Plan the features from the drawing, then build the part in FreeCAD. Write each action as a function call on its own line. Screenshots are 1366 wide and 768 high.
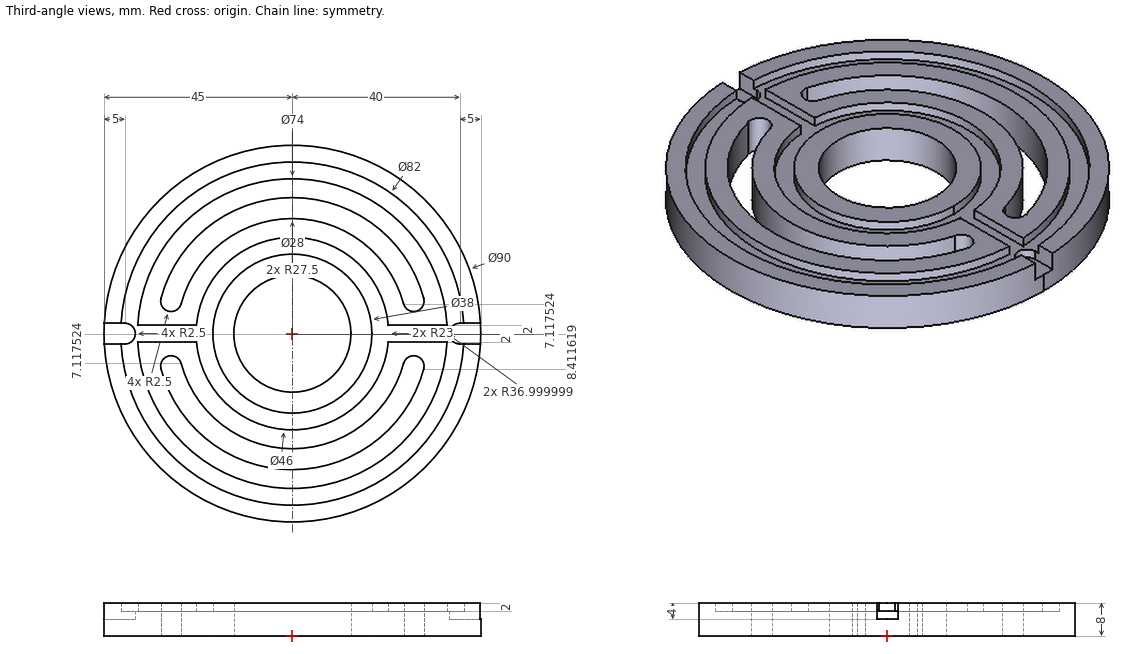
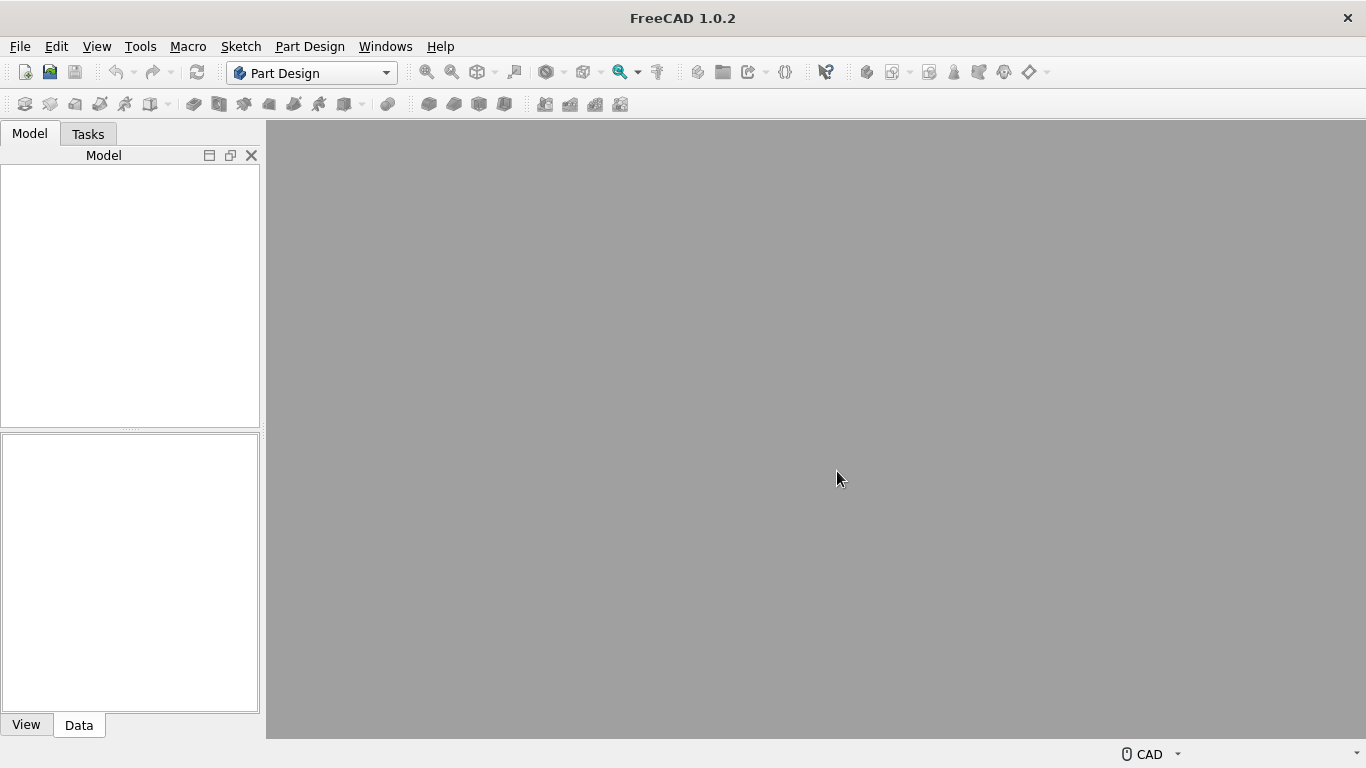
key(ctrl+n)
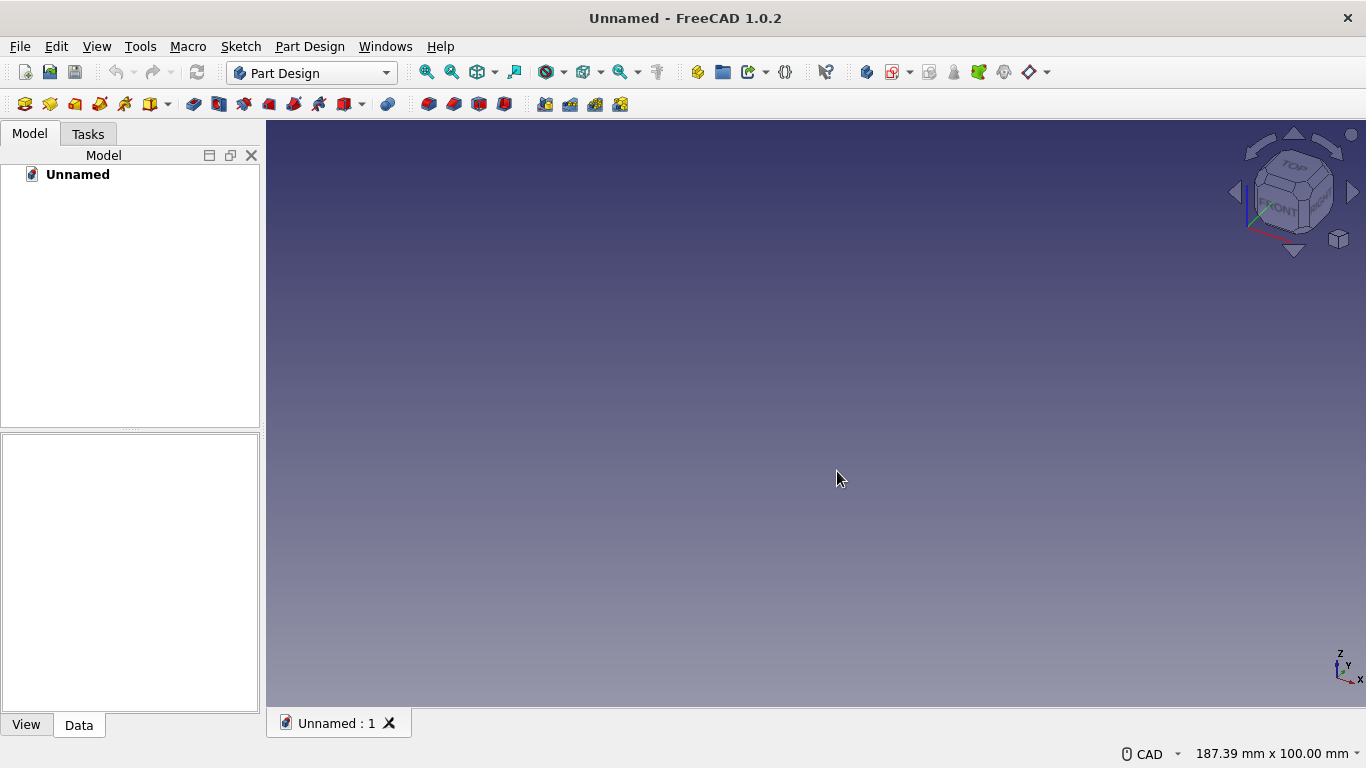
click(892, 72)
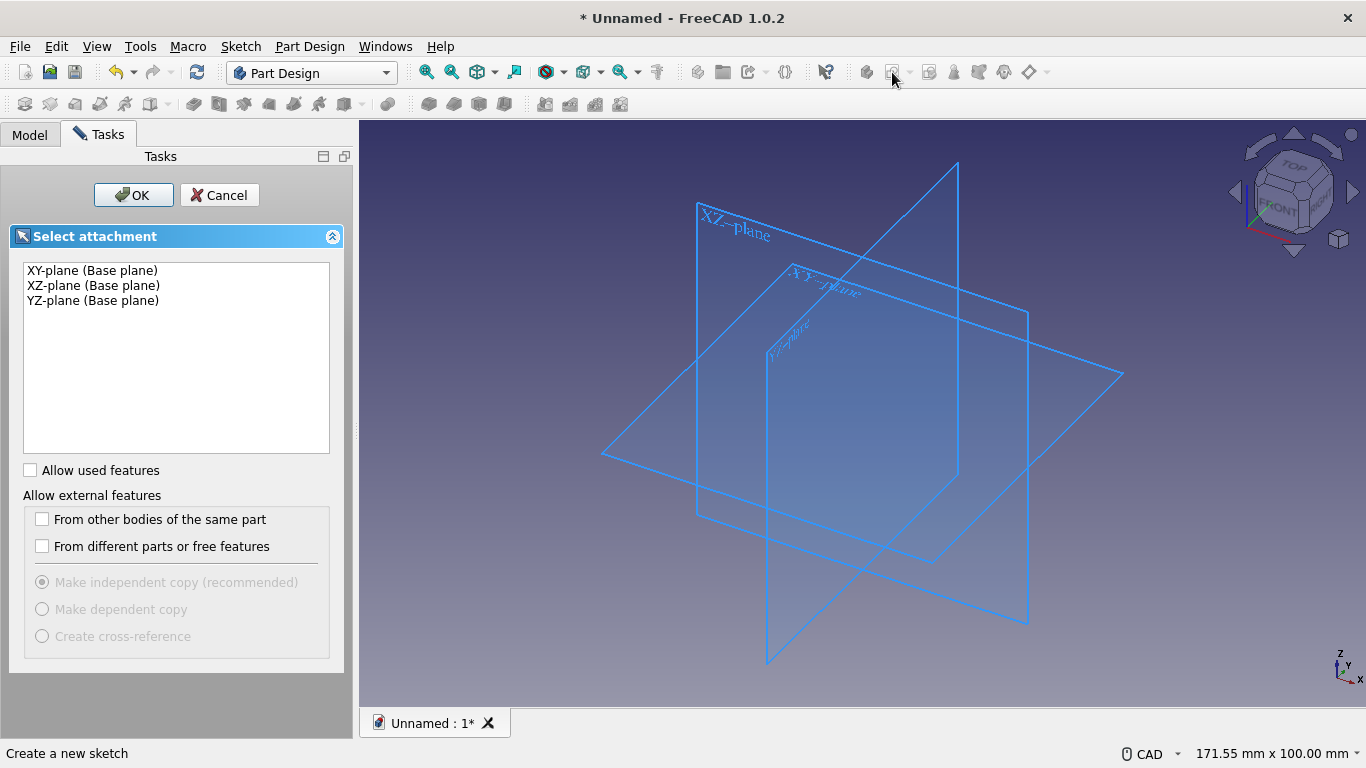
click(84, 270)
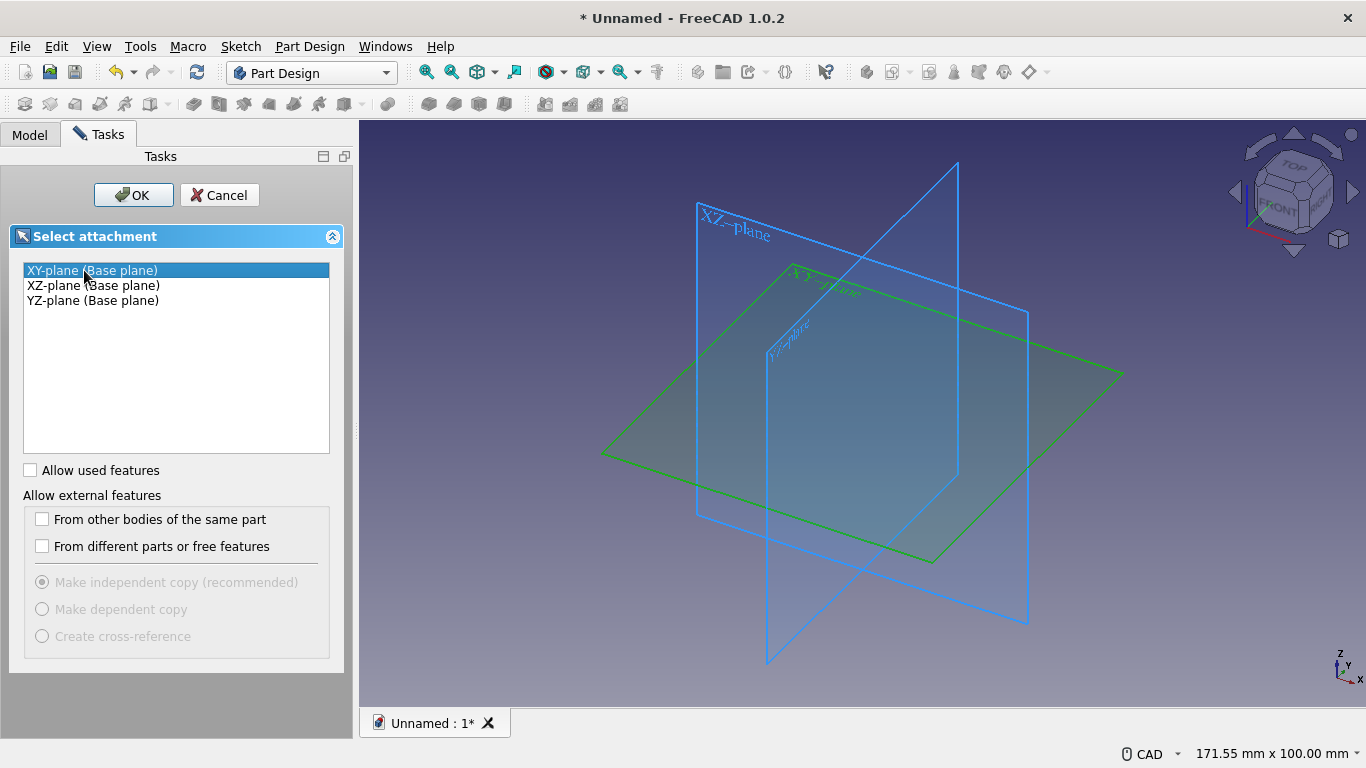
click(134, 195)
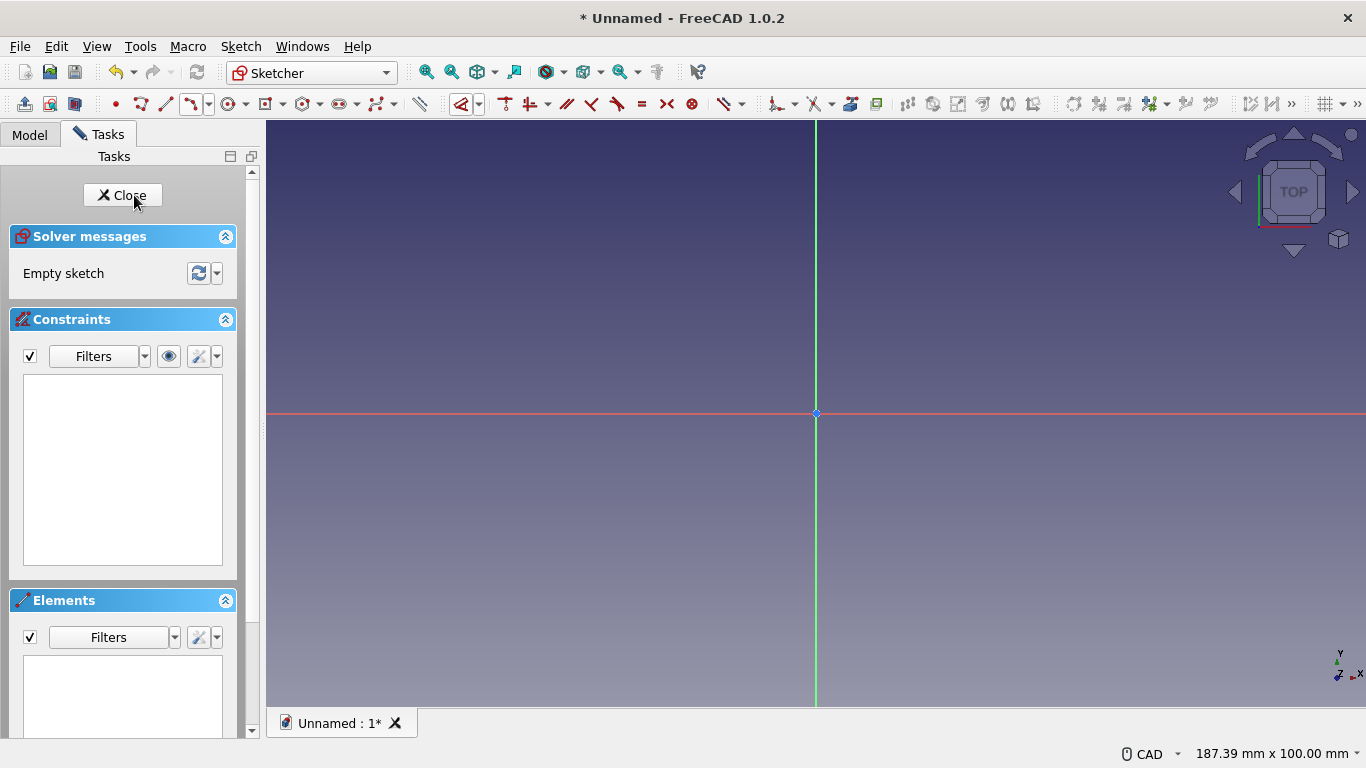
scroll(608, 414, down, 2)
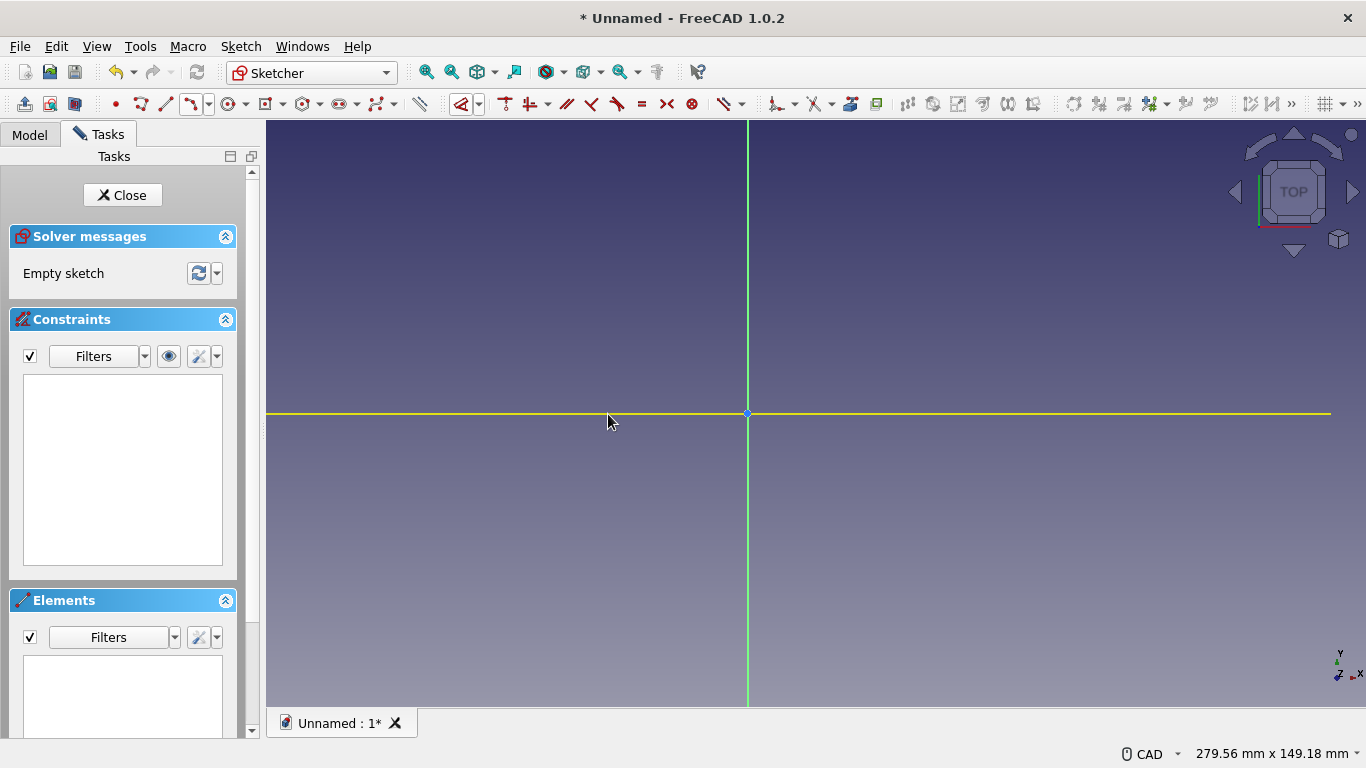
click(228, 104)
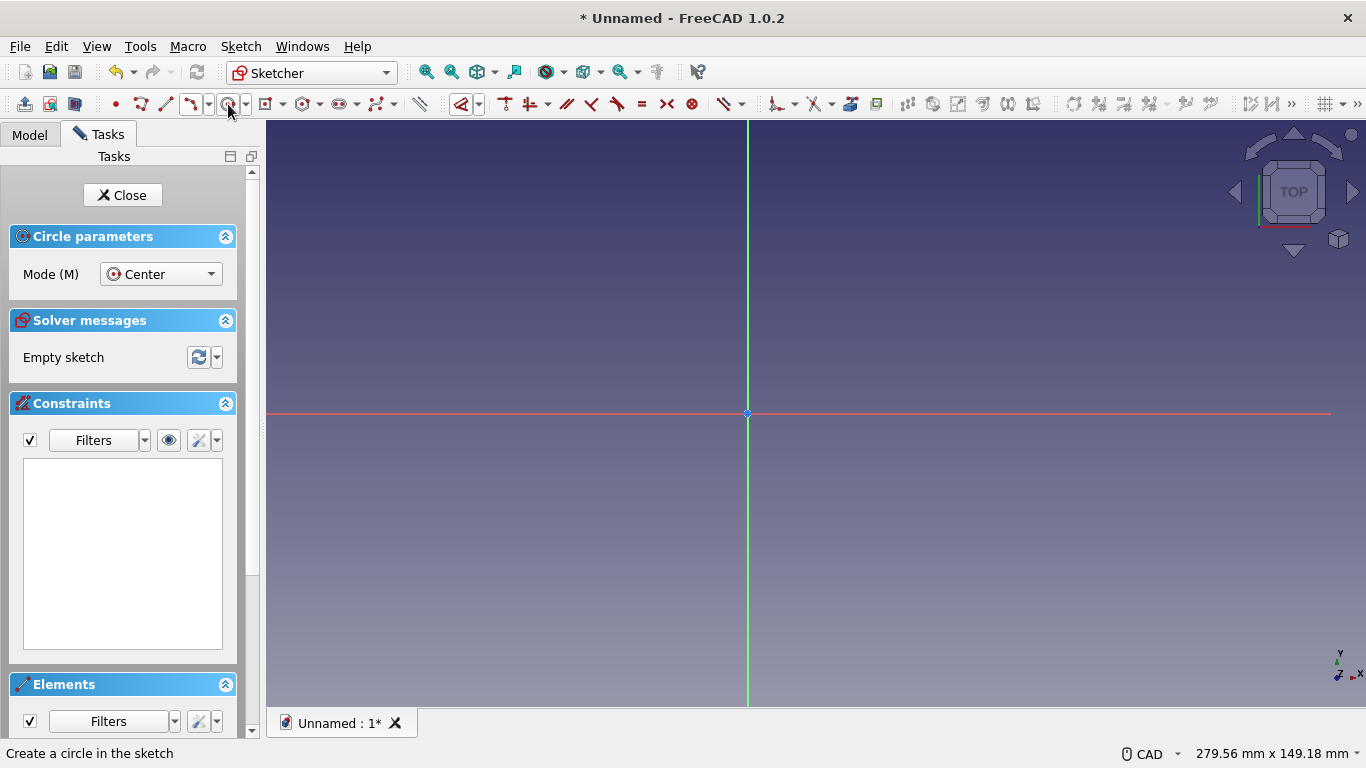
click(748, 414)
move(873, 289)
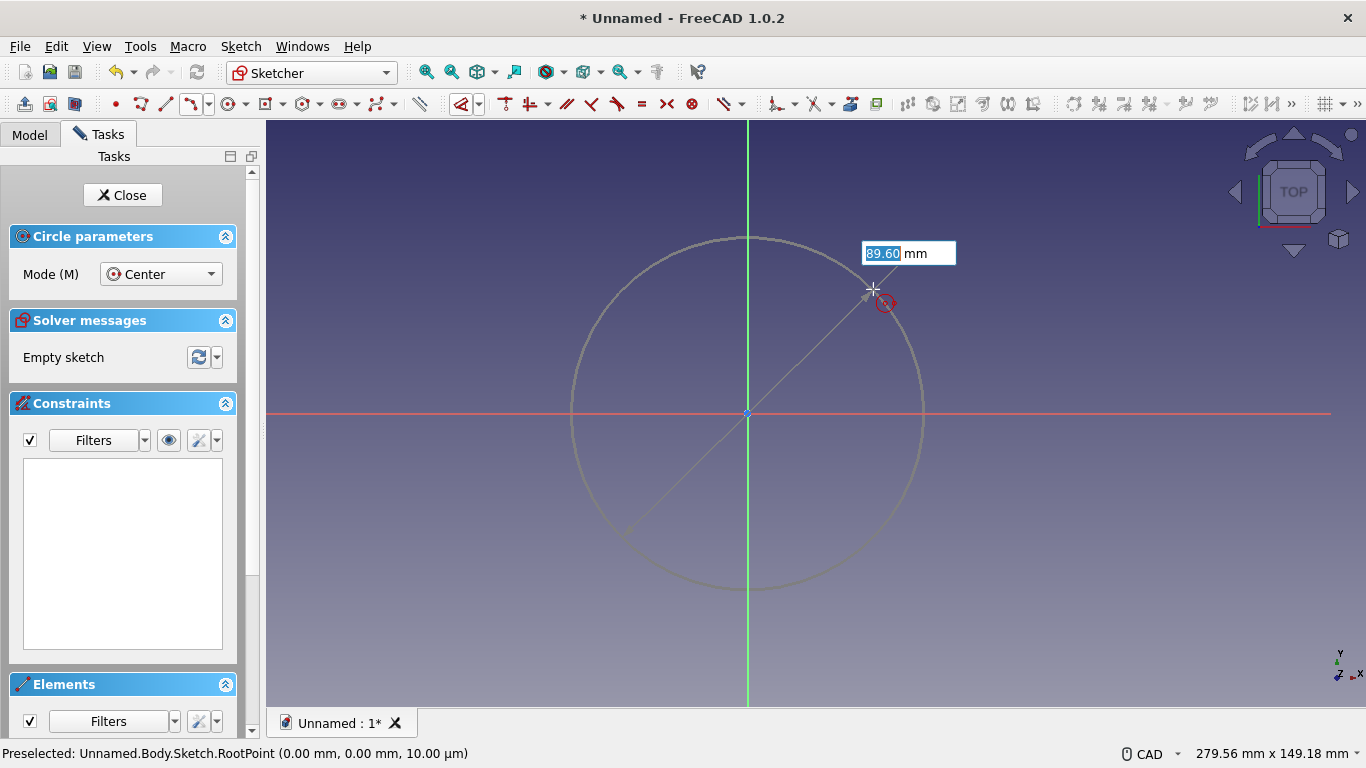
text(90)
key(Return)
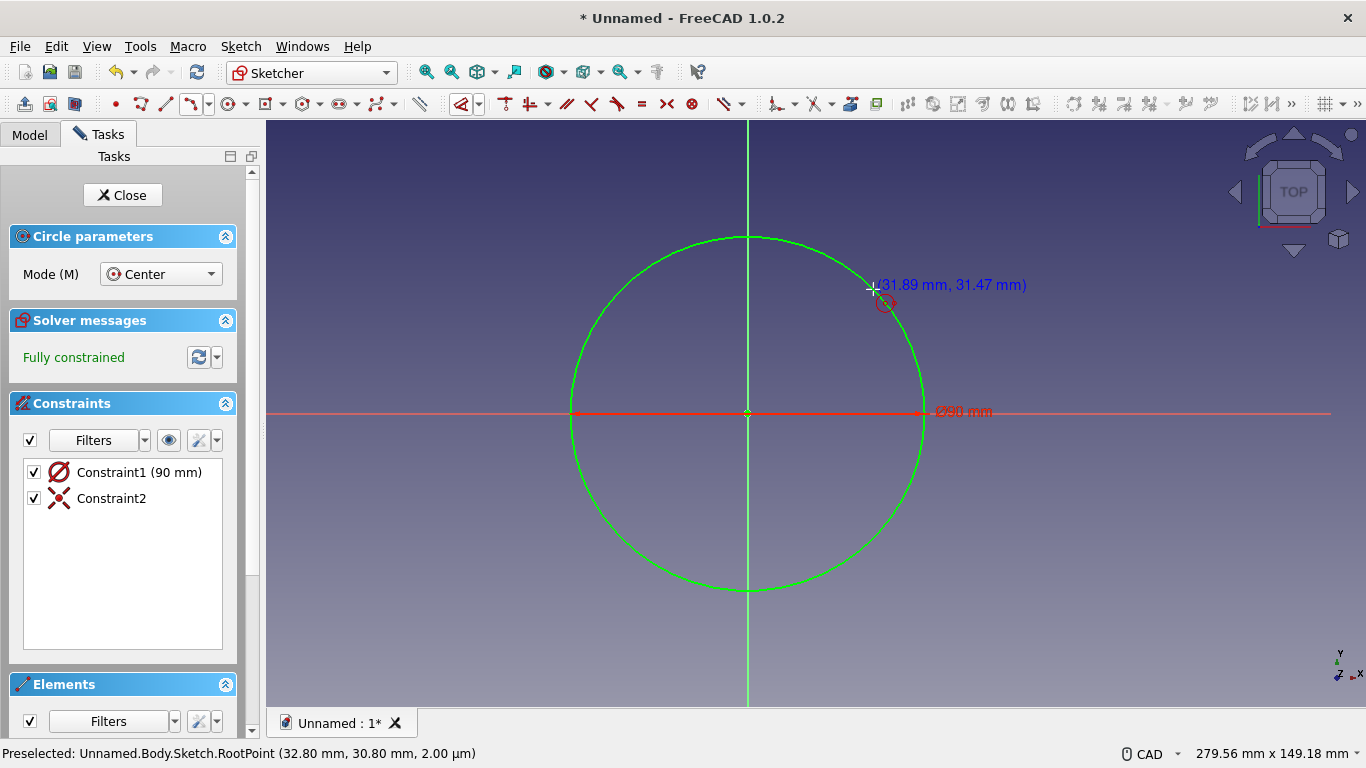
click(748, 414)
move(786, 375)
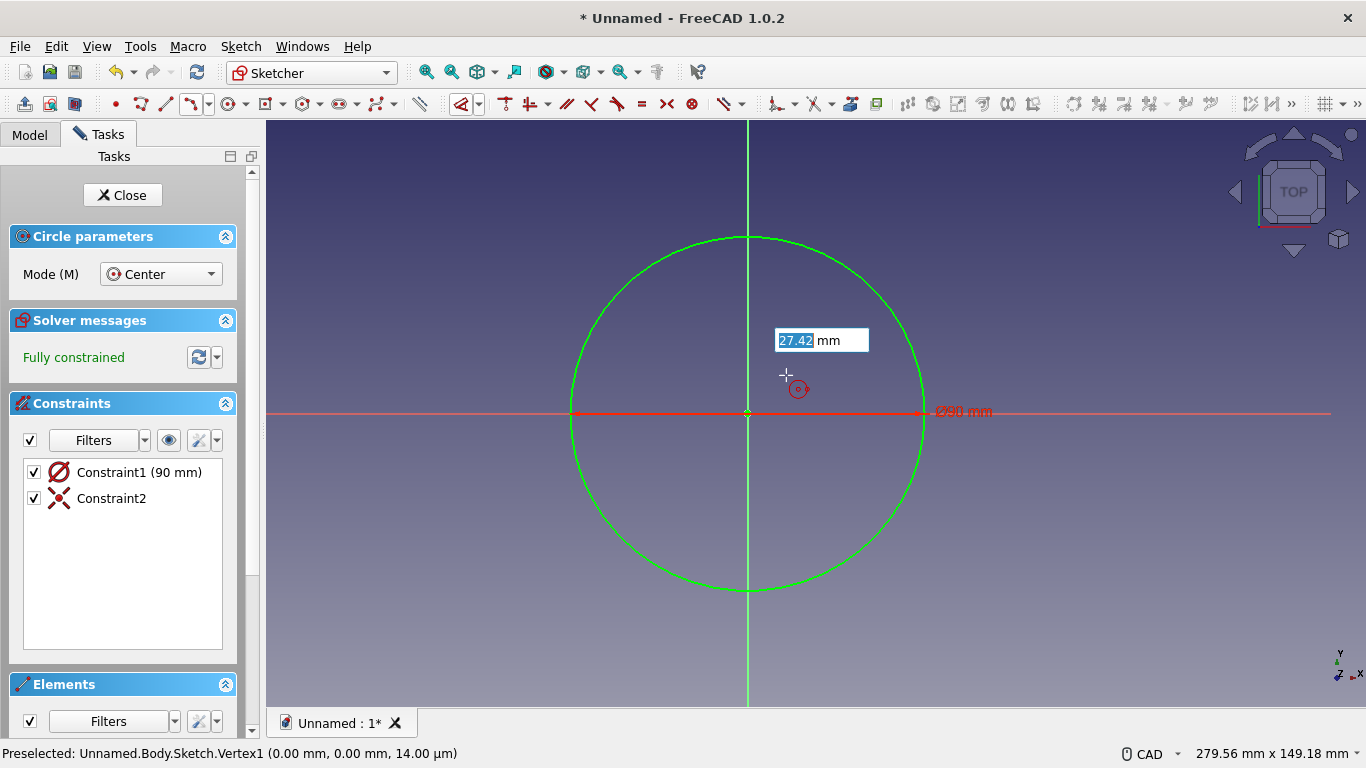
text(28)
key(Return)
key(Escape)